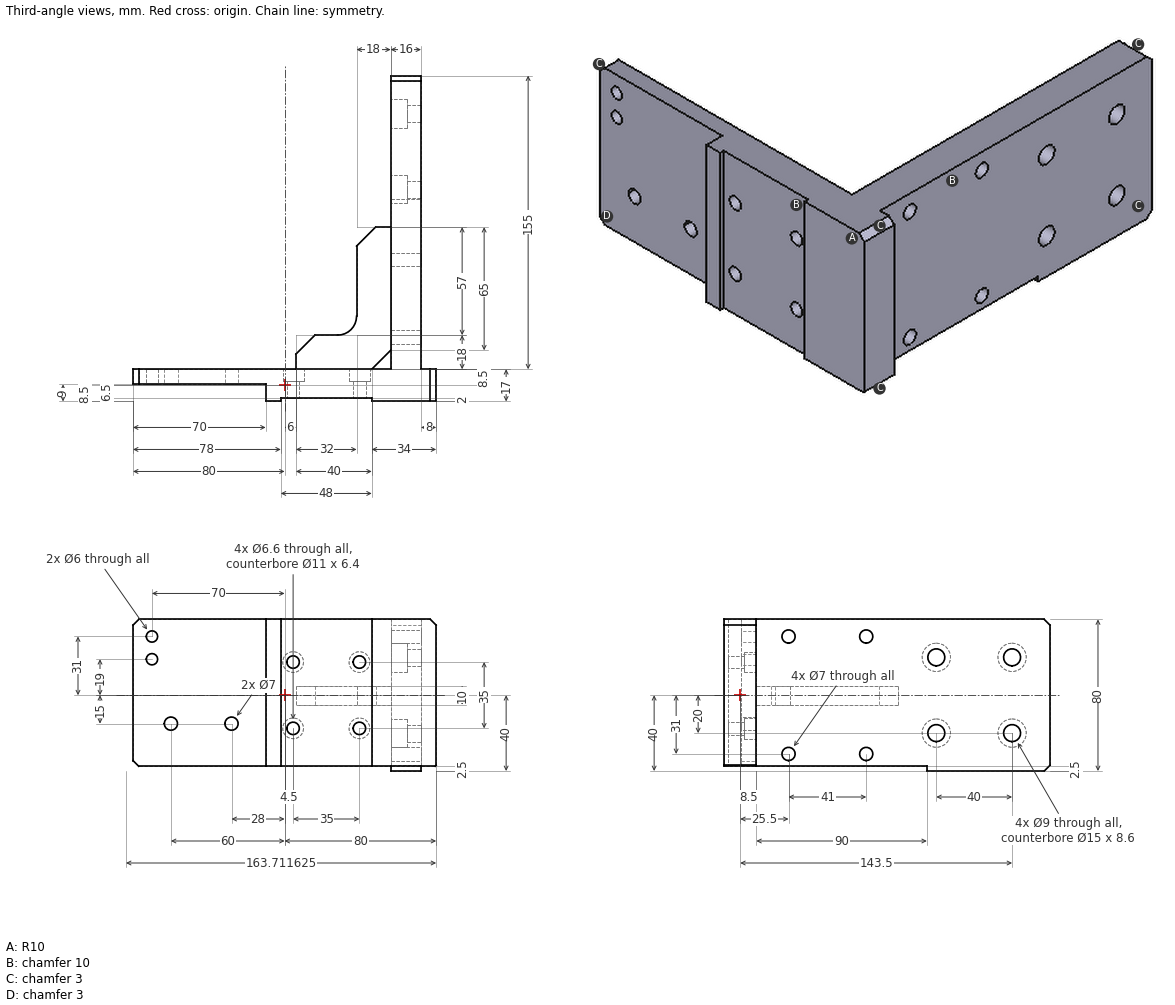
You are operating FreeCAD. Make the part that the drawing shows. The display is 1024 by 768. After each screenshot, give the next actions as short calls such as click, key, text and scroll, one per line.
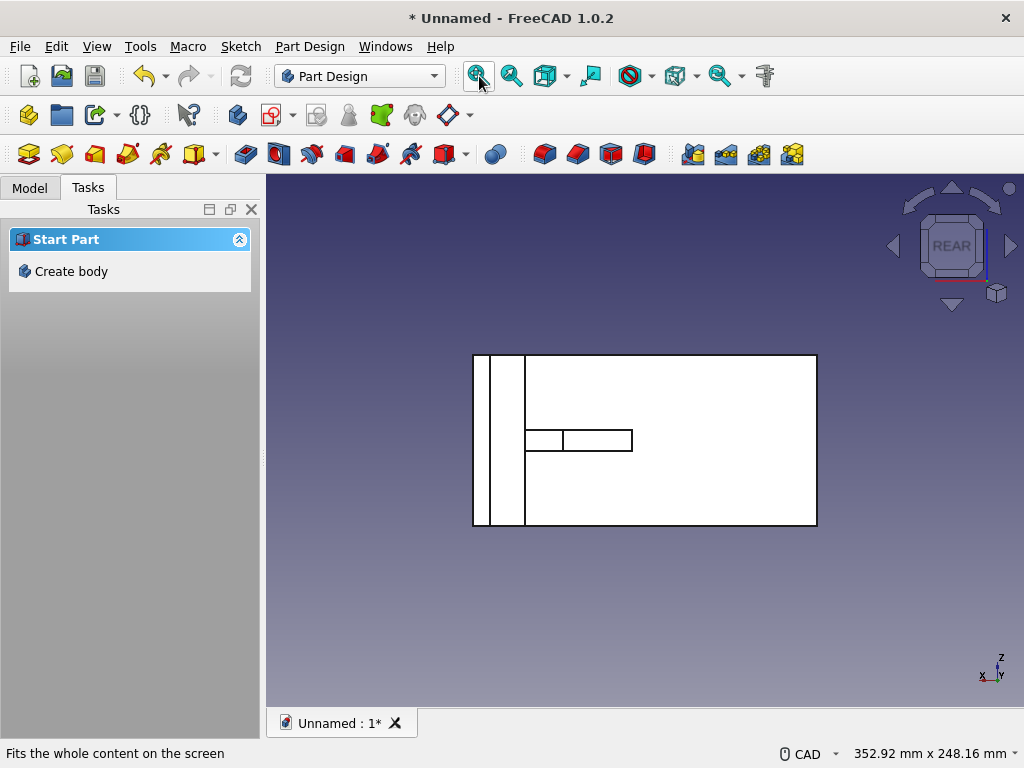
scroll(563, 440, up, 4)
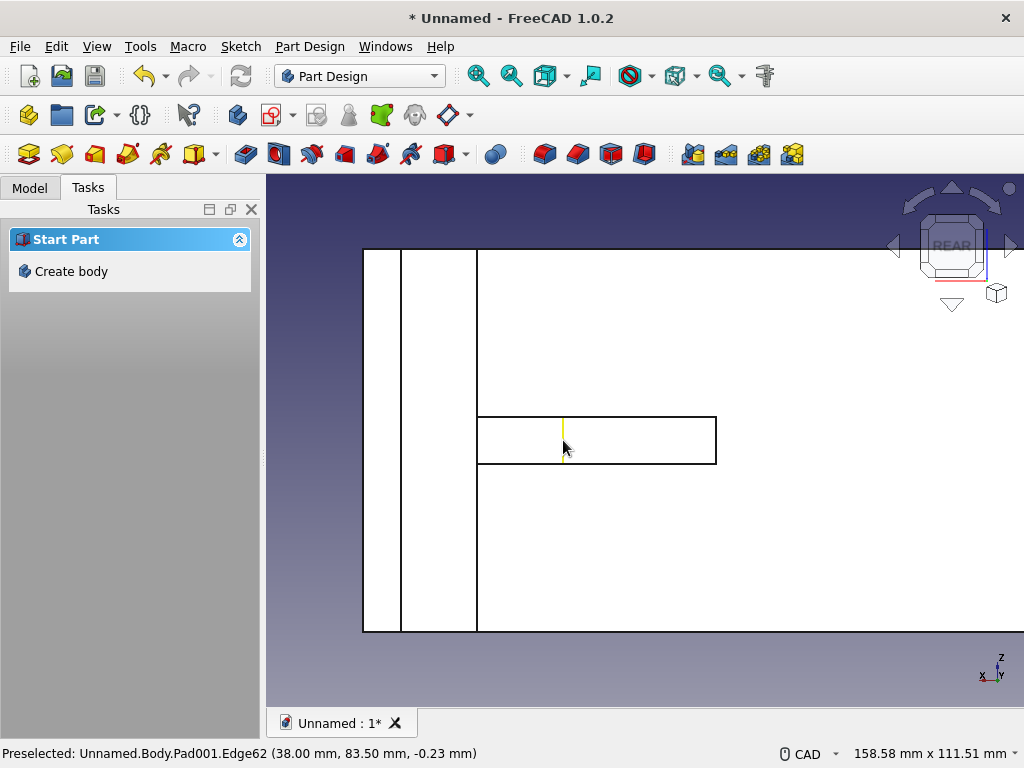
click(479, 76)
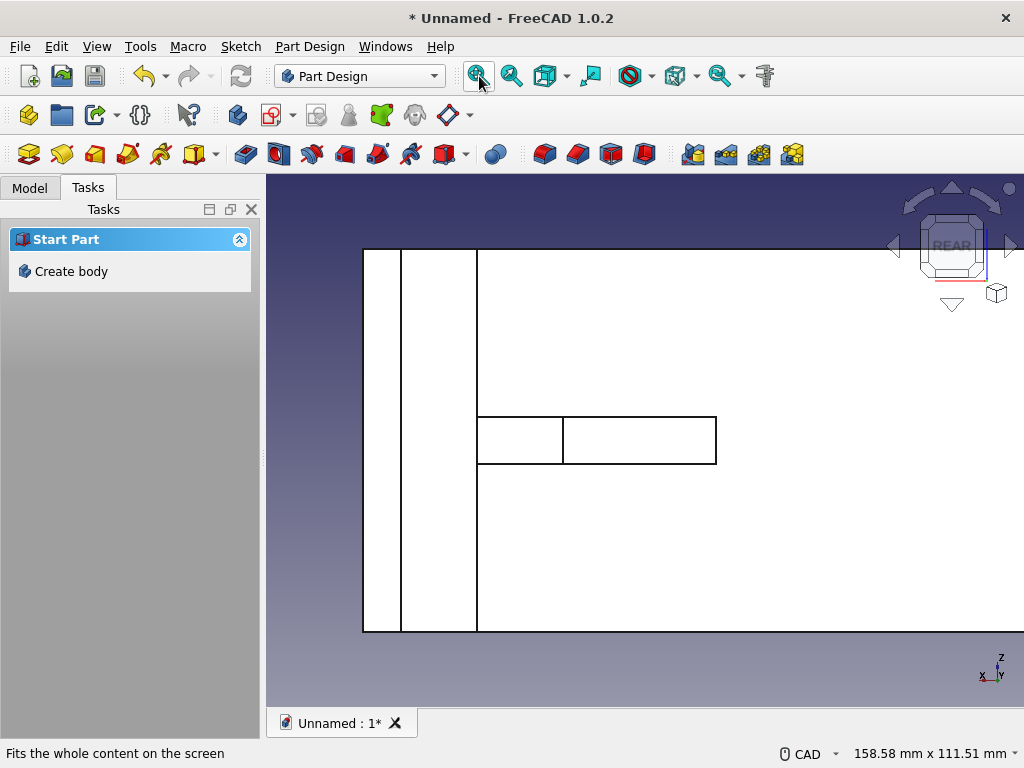
key(6)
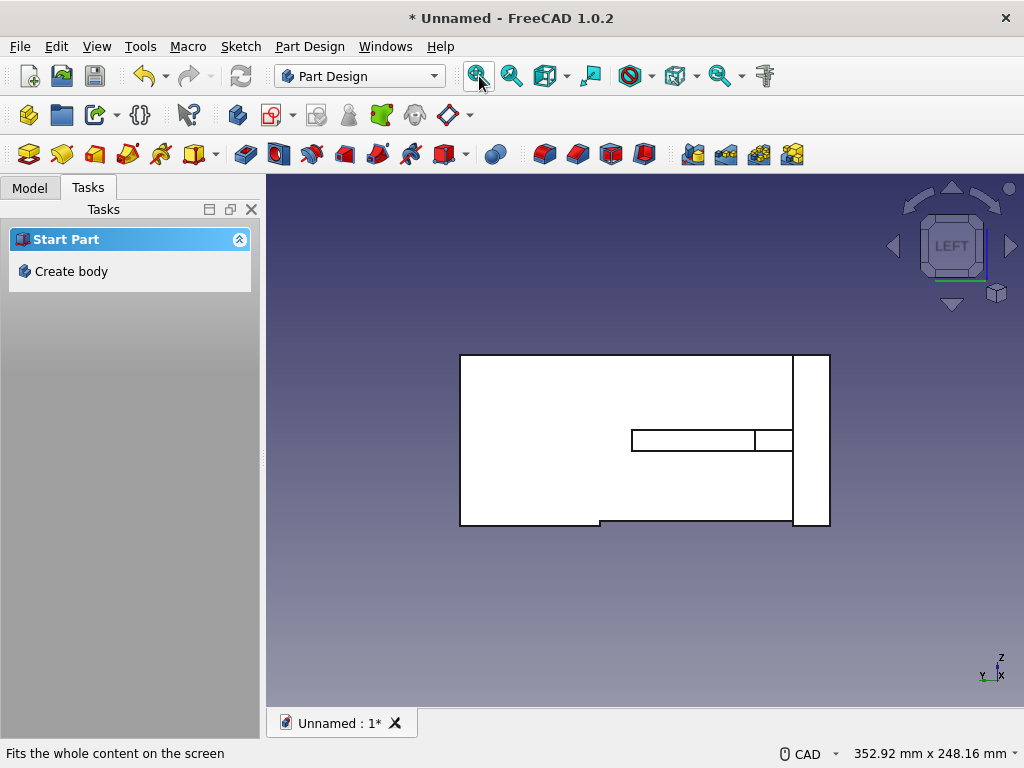
scroll(755, 439, up, 4)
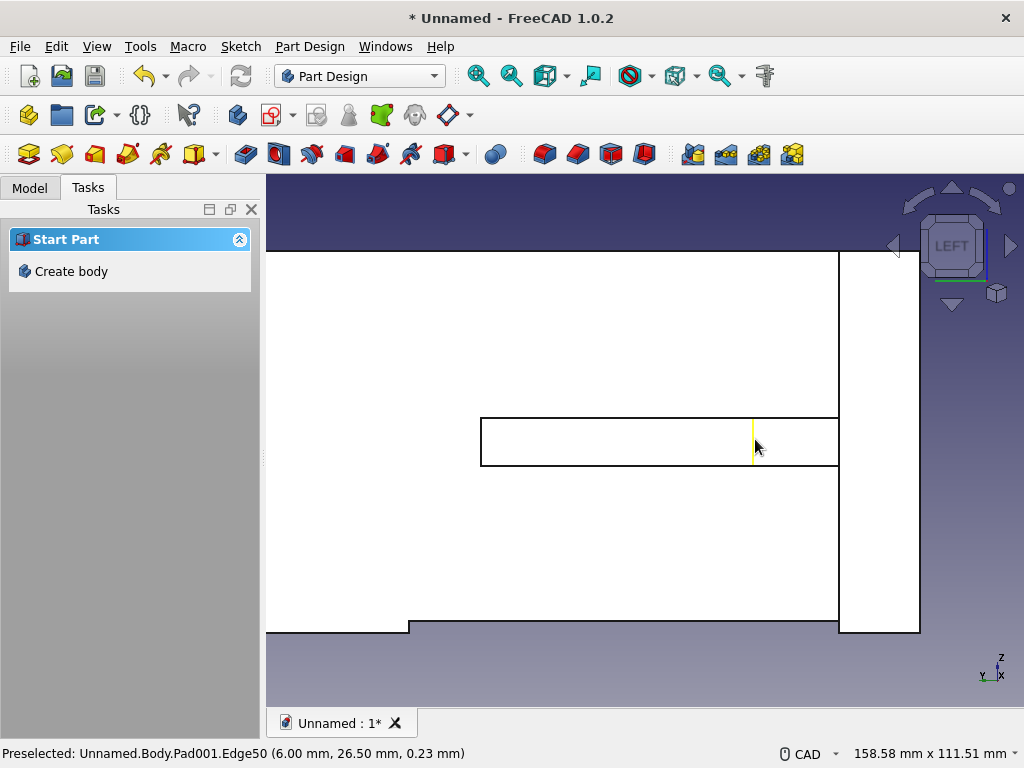
key(v)
key(f)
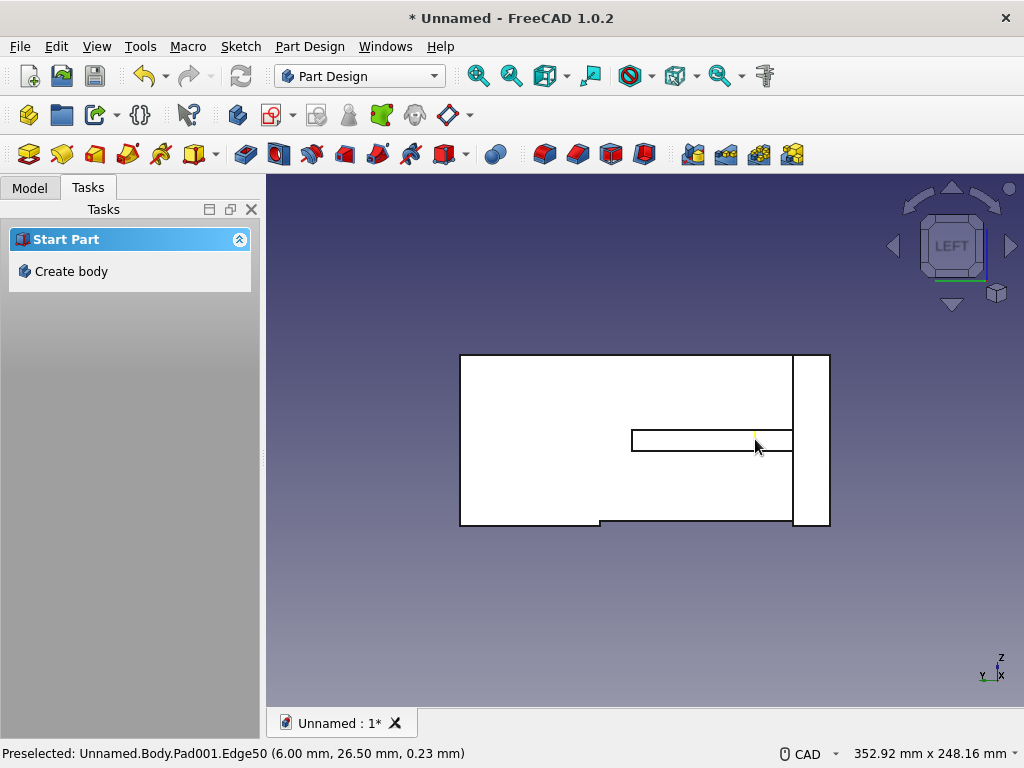
key(v)
key(3)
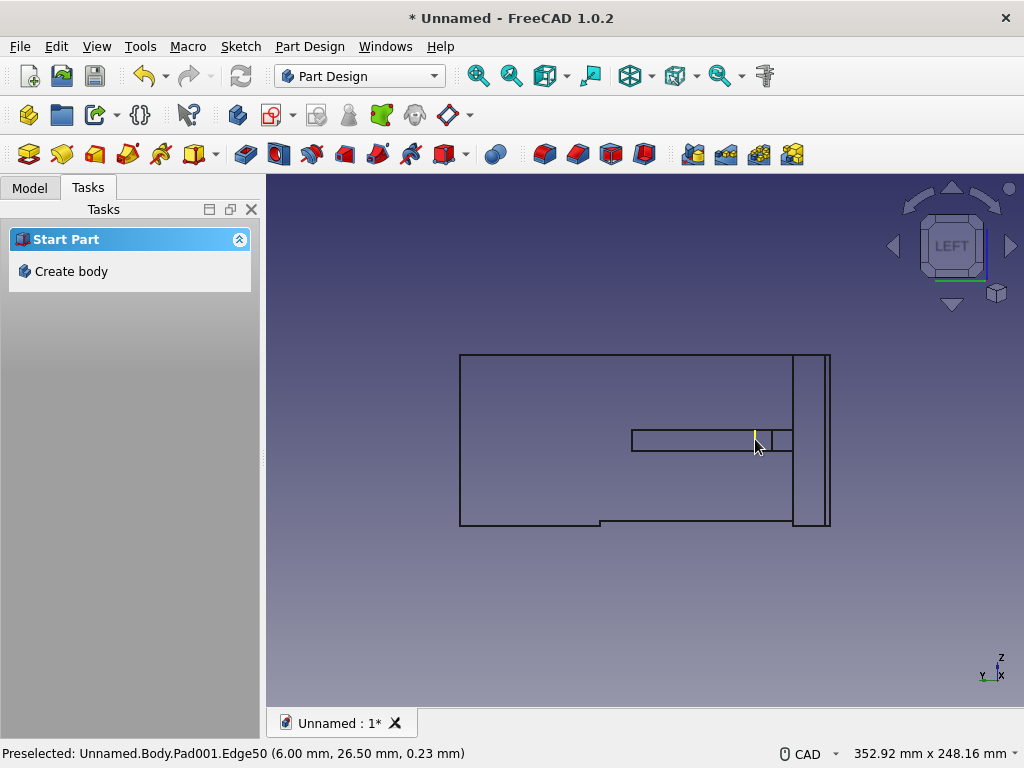
key(0)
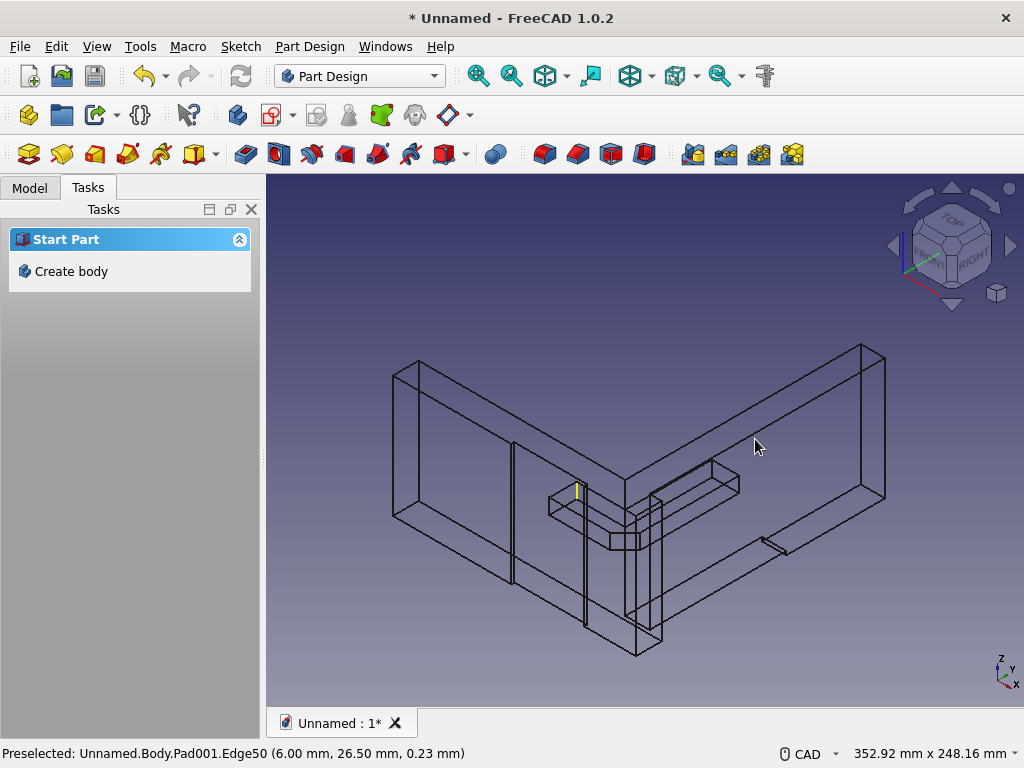
scroll(625, 518, up, 4)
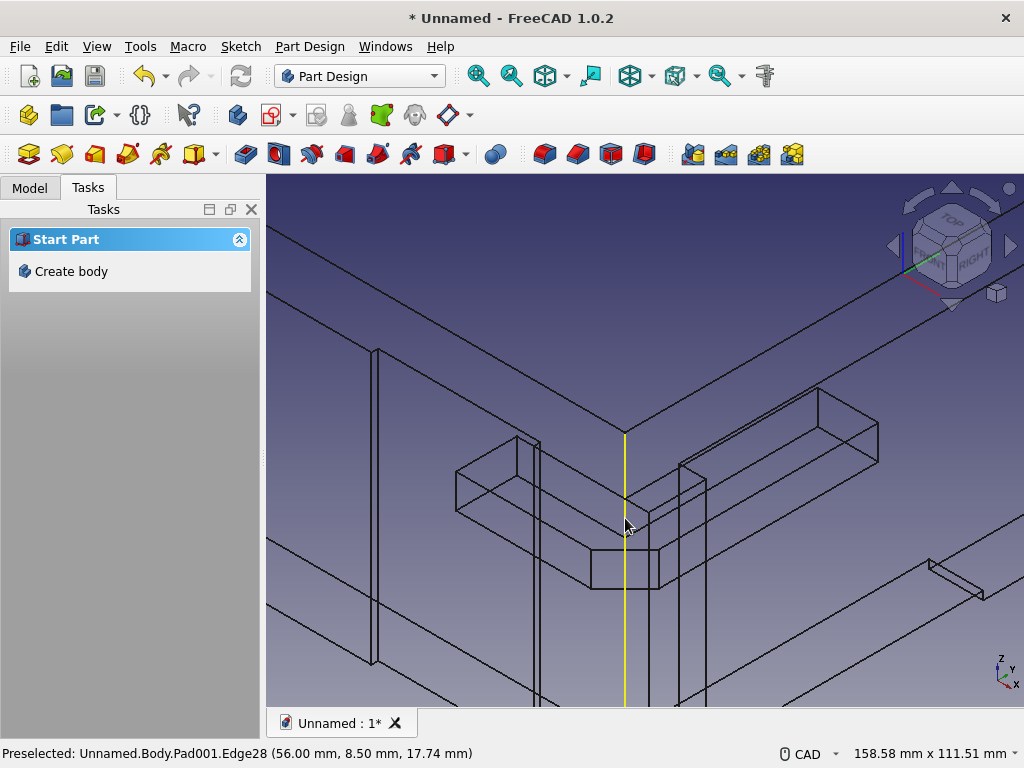
click(479, 76)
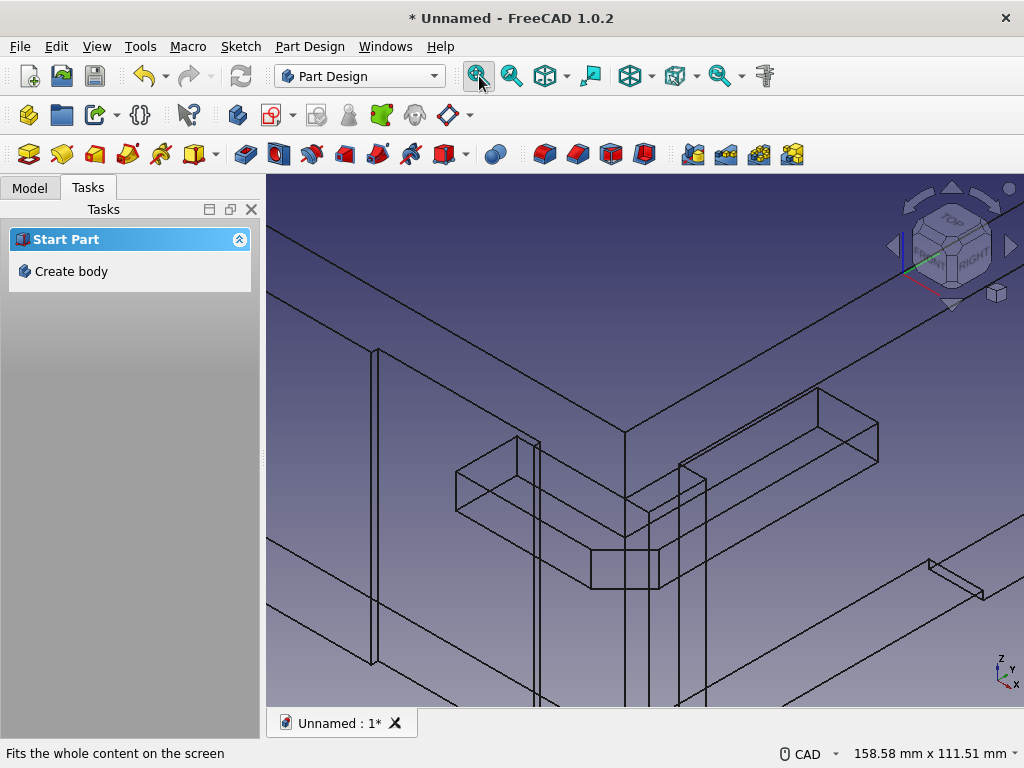
key(2)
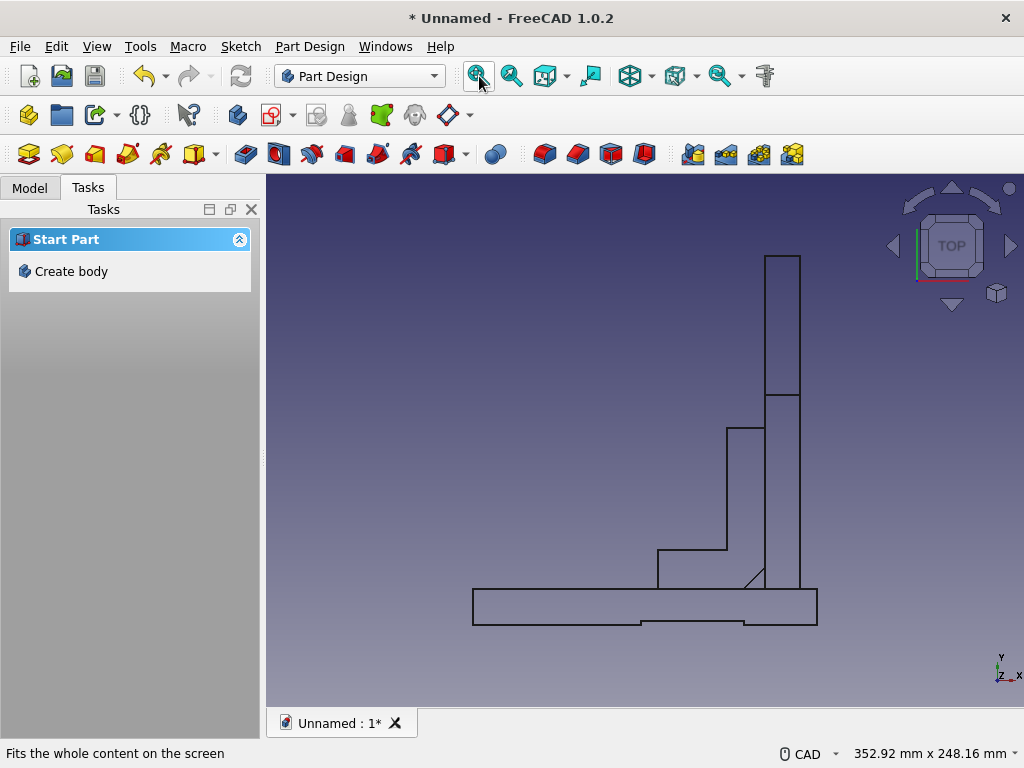
scroll(727, 549, up, 4)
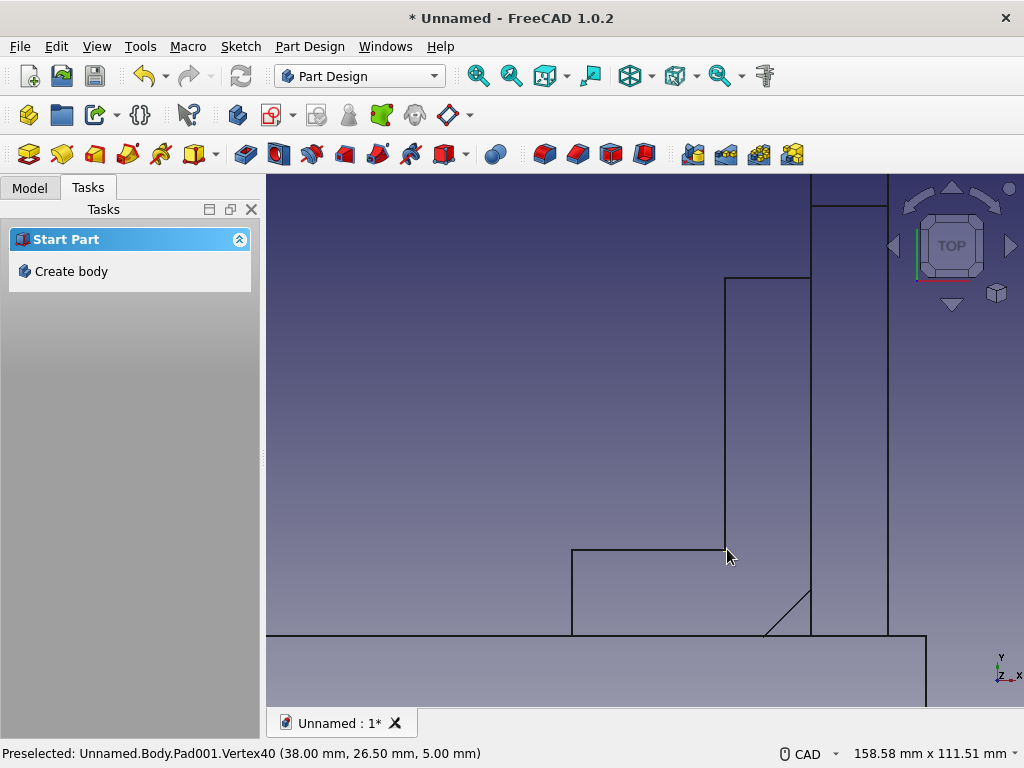
click(479, 76)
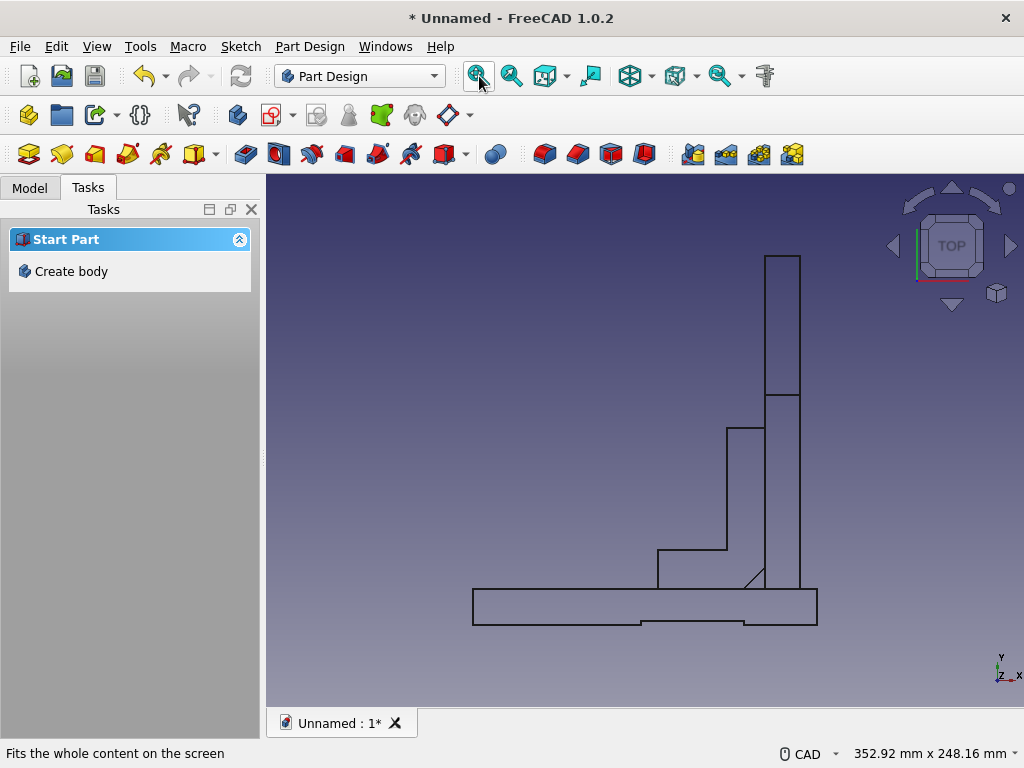
key(1)